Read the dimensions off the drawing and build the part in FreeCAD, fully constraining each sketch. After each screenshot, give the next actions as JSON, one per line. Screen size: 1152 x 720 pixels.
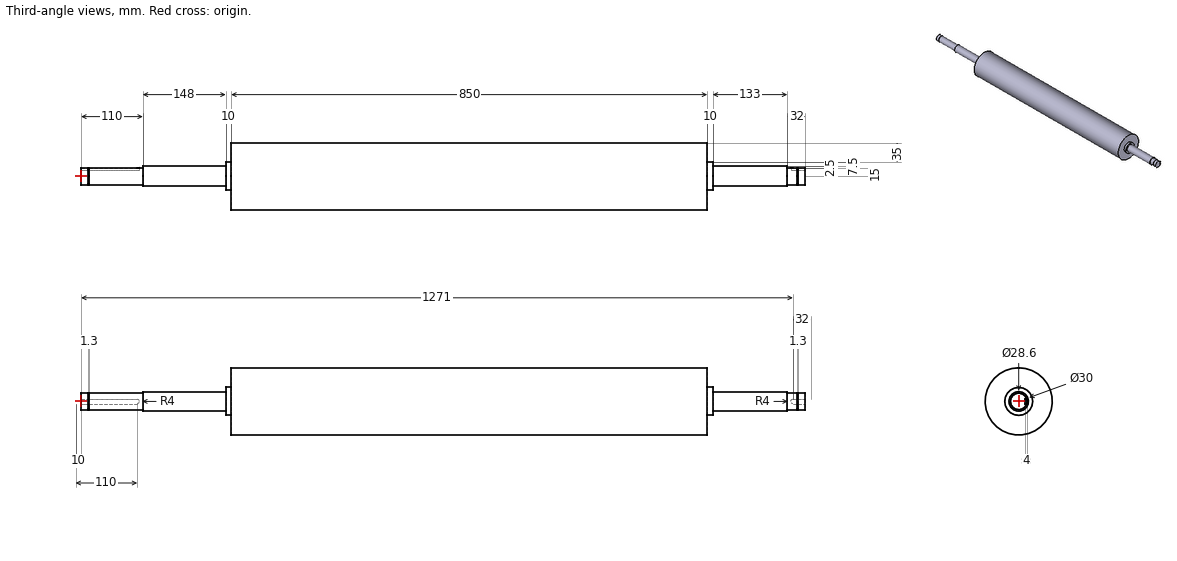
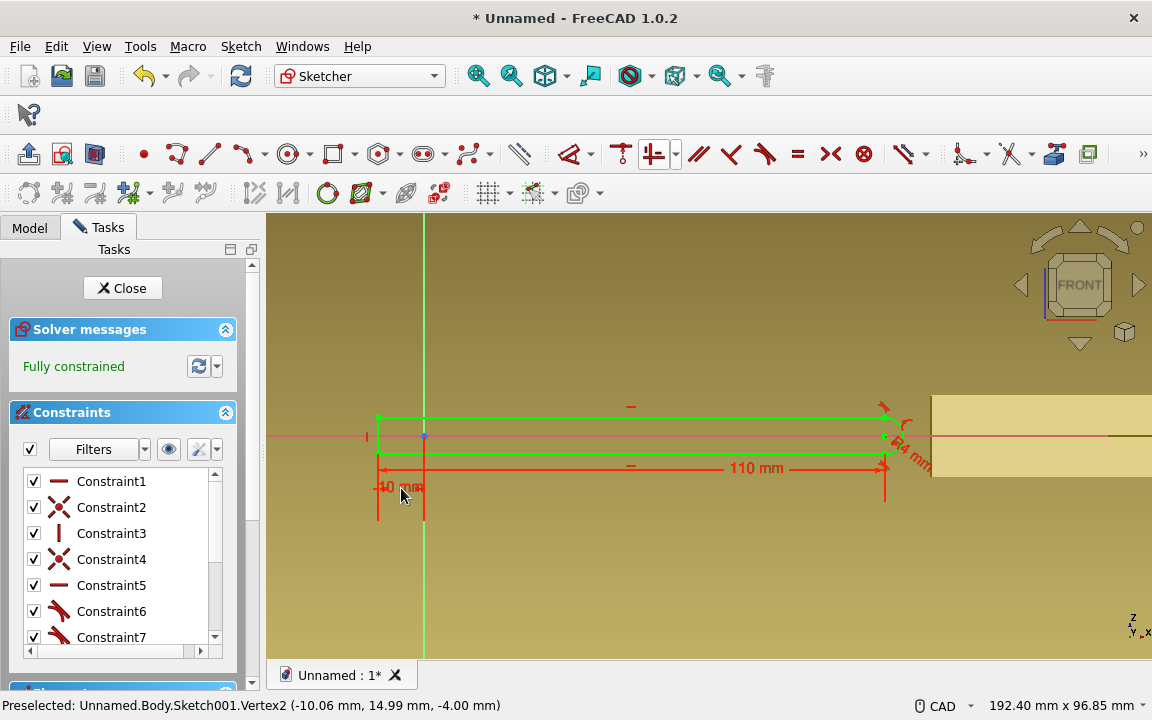
{"action": "left_click", "coordinate": [123, 288]}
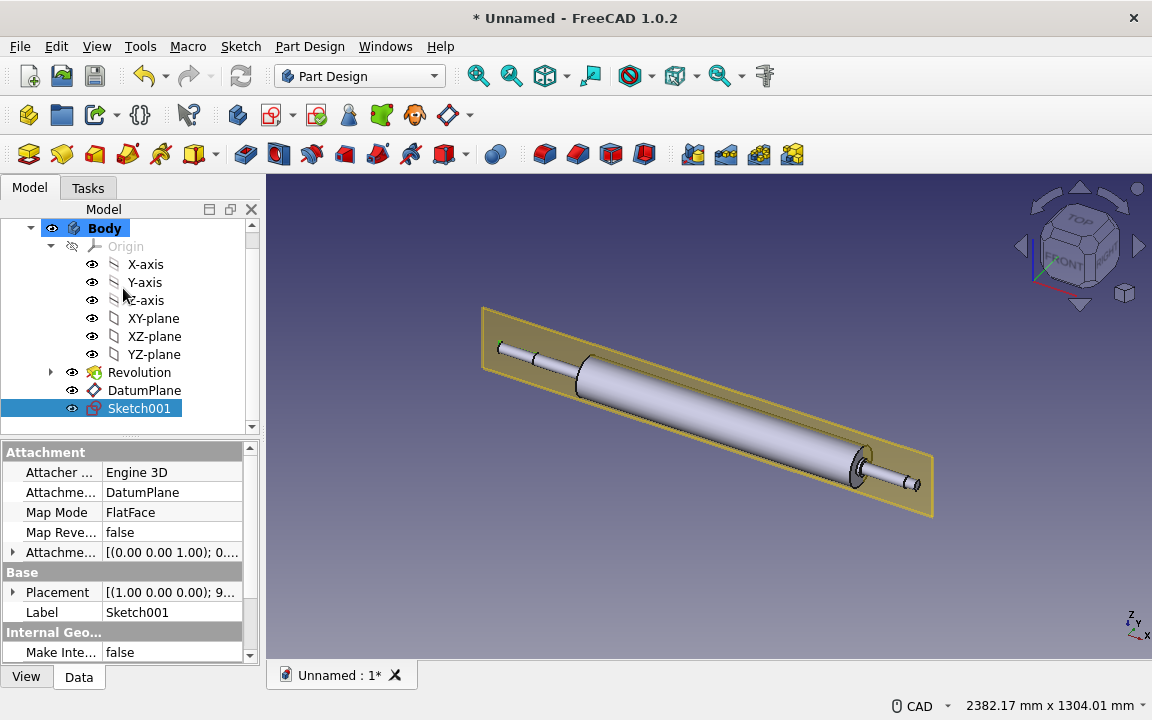
{"action": "left_click", "coordinate": [246, 154]}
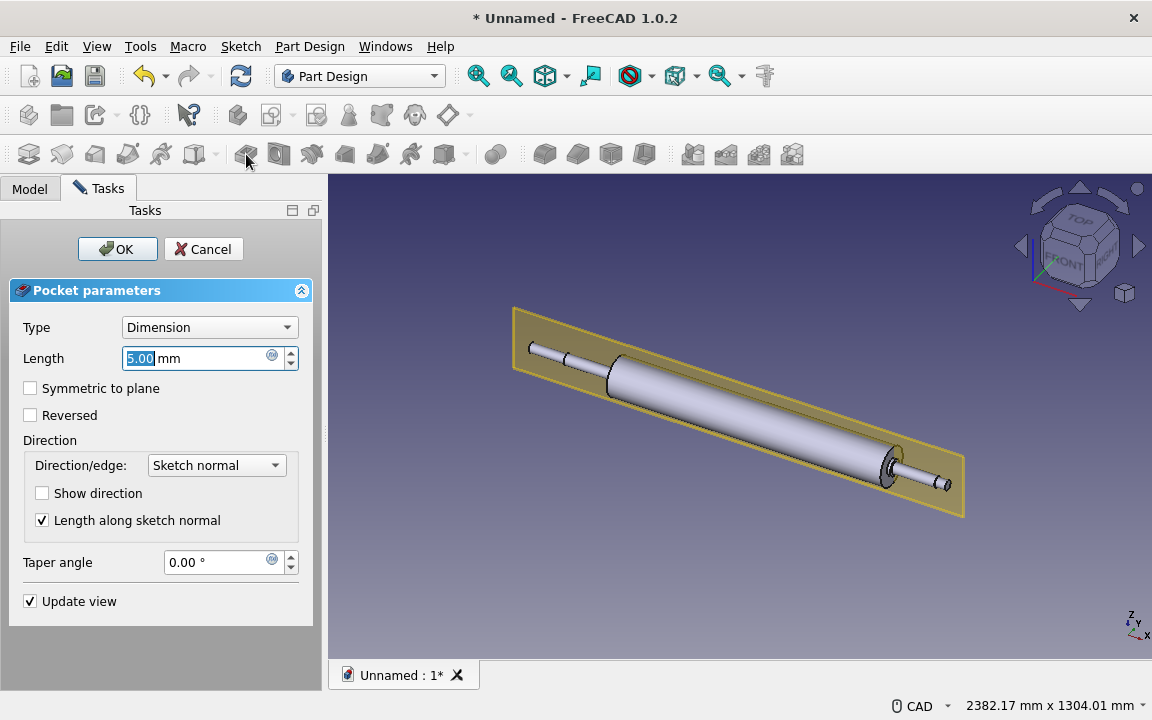
{"action": "type", "text": "4"}
{"action": "key", "text": "Tab"}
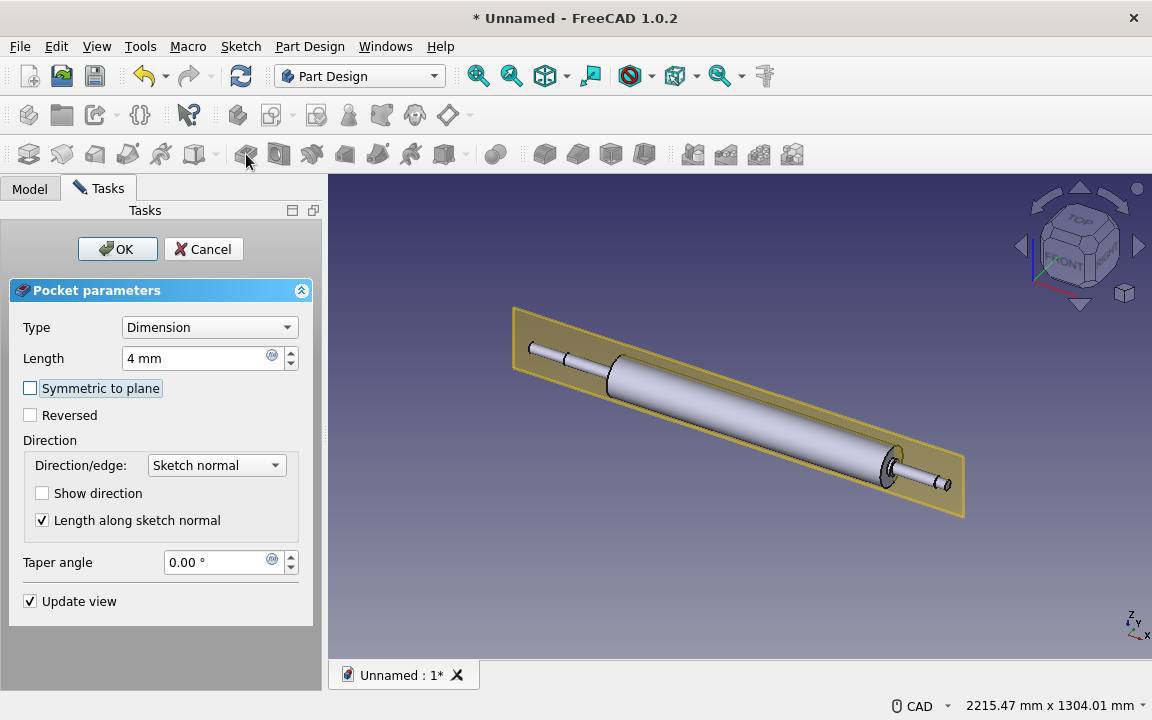
{"action": "left_click", "coordinate": [31, 415]}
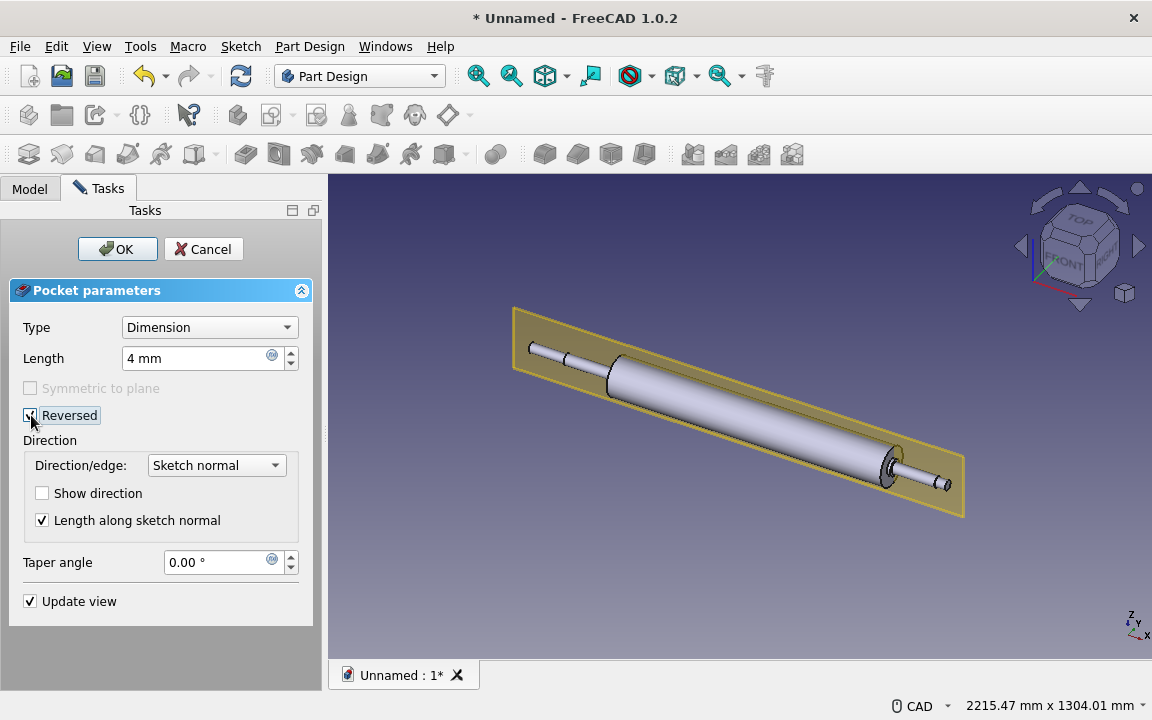
{"action": "left_click", "coordinate": [118, 249]}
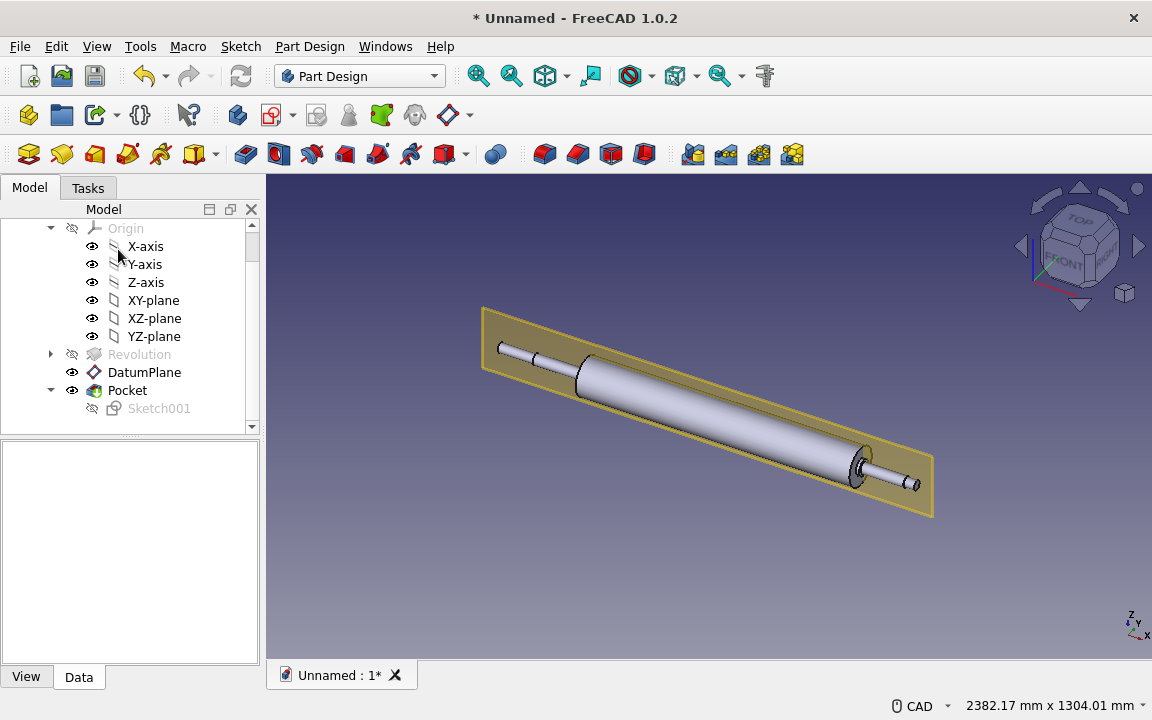
{"action": "left_click", "coordinate": [117, 372]}
{"action": "key", "text": "space"}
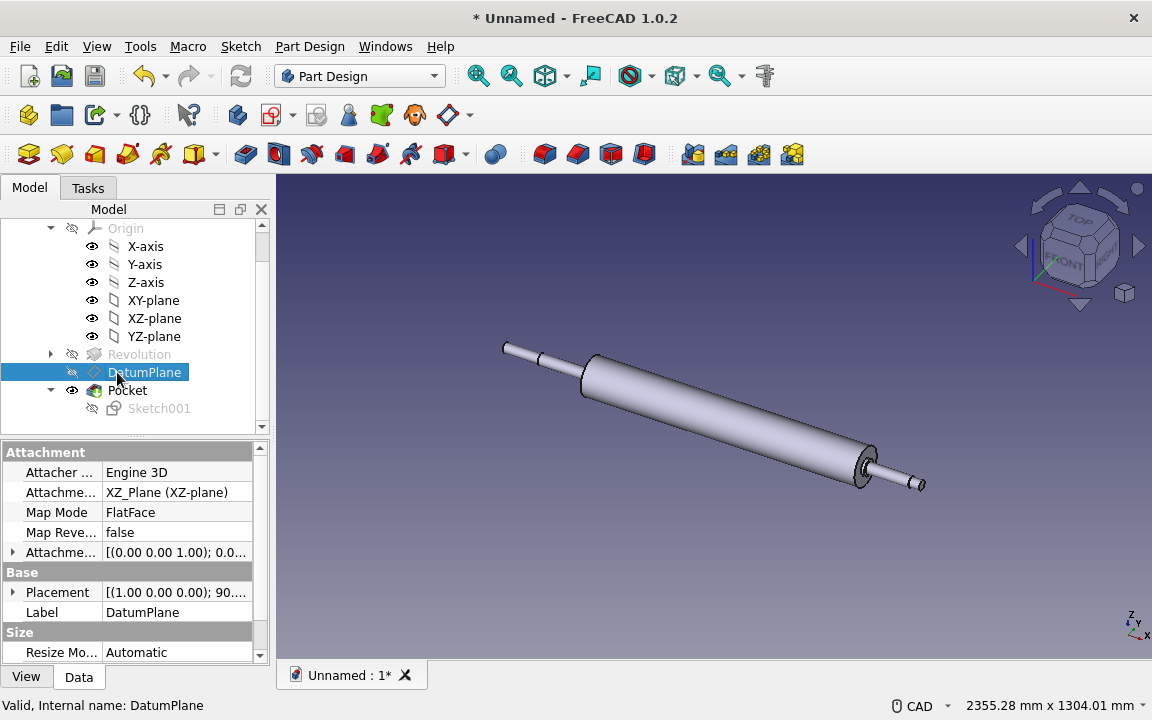
{"action": "left_click", "coordinate": [137, 336]}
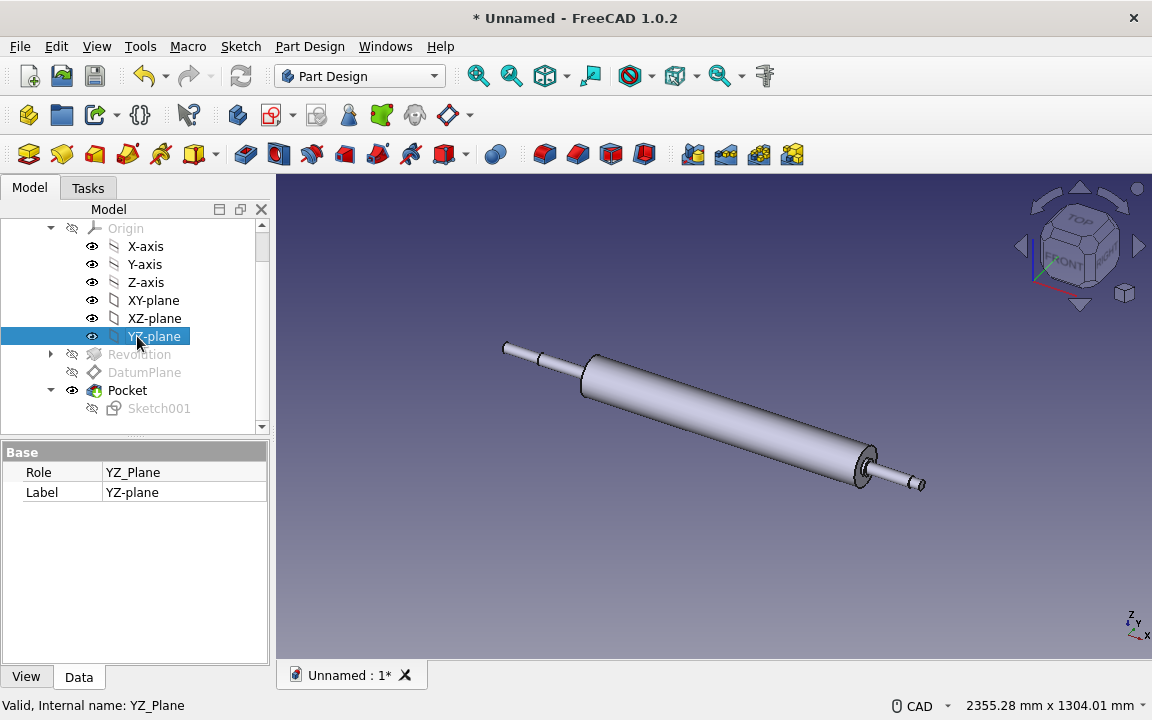
{"action": "left_click", "coordinate": [448, 116]}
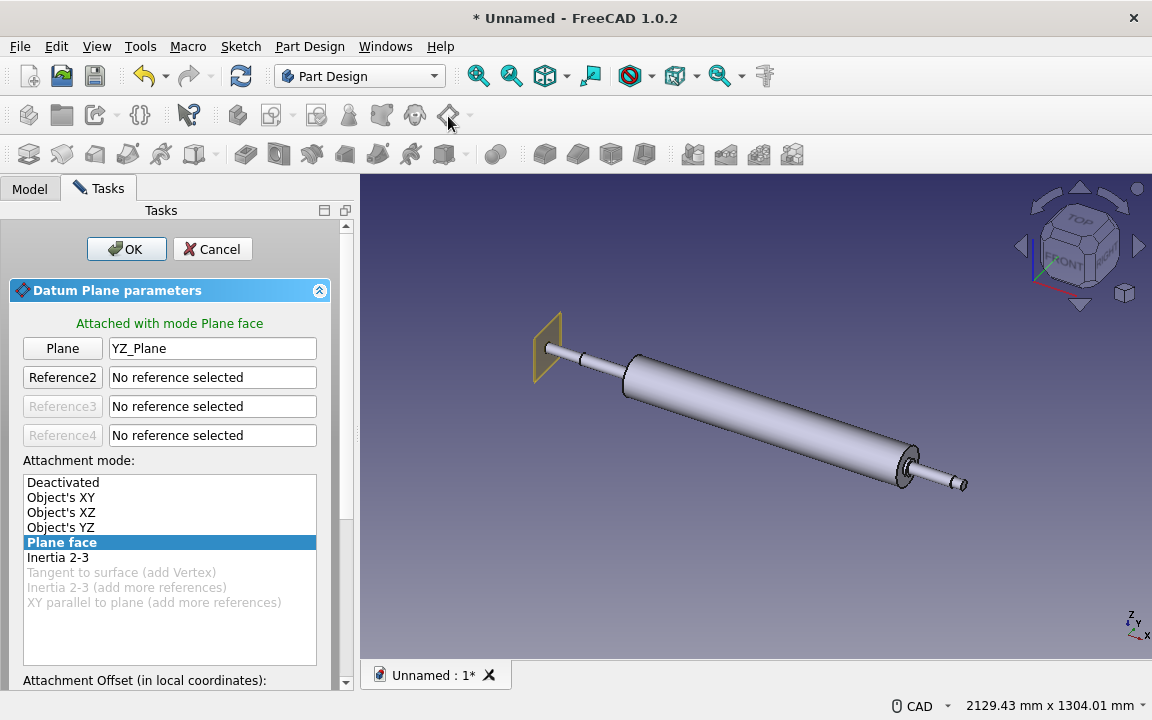
{"action": "scroll", "coordinate": [346, 455], "scroll_direction": "down", "scroll_amount": 3}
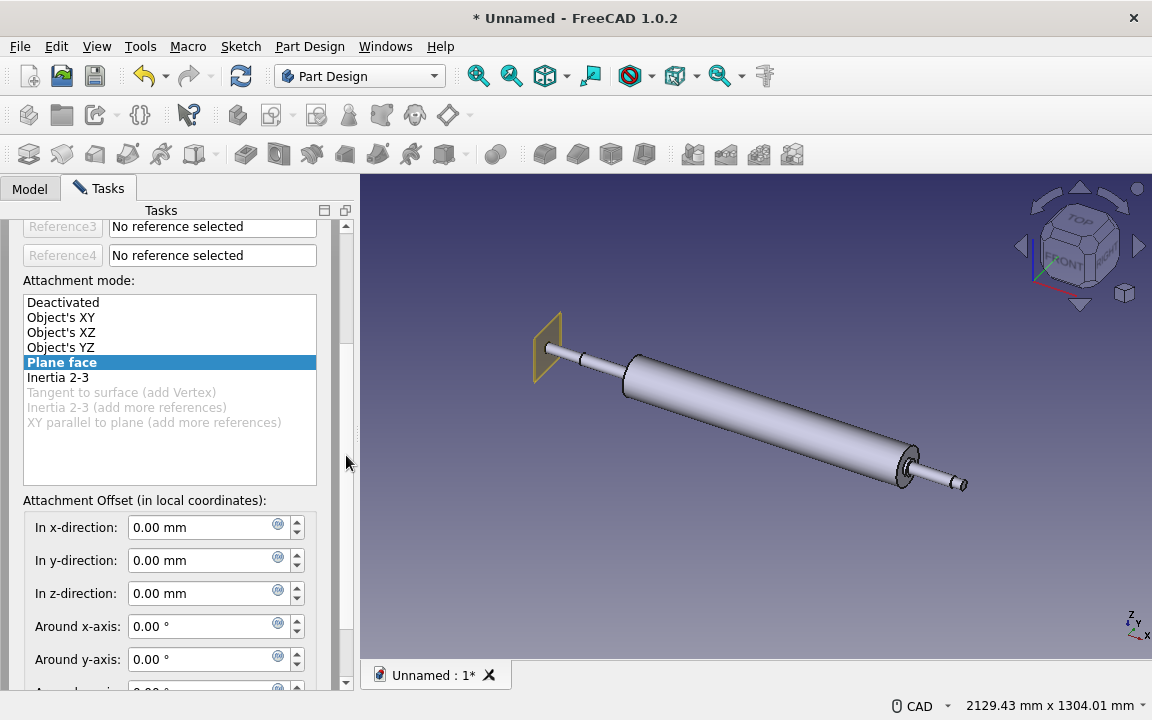
{"action": "triple_click", "coordinate": [210, 594]}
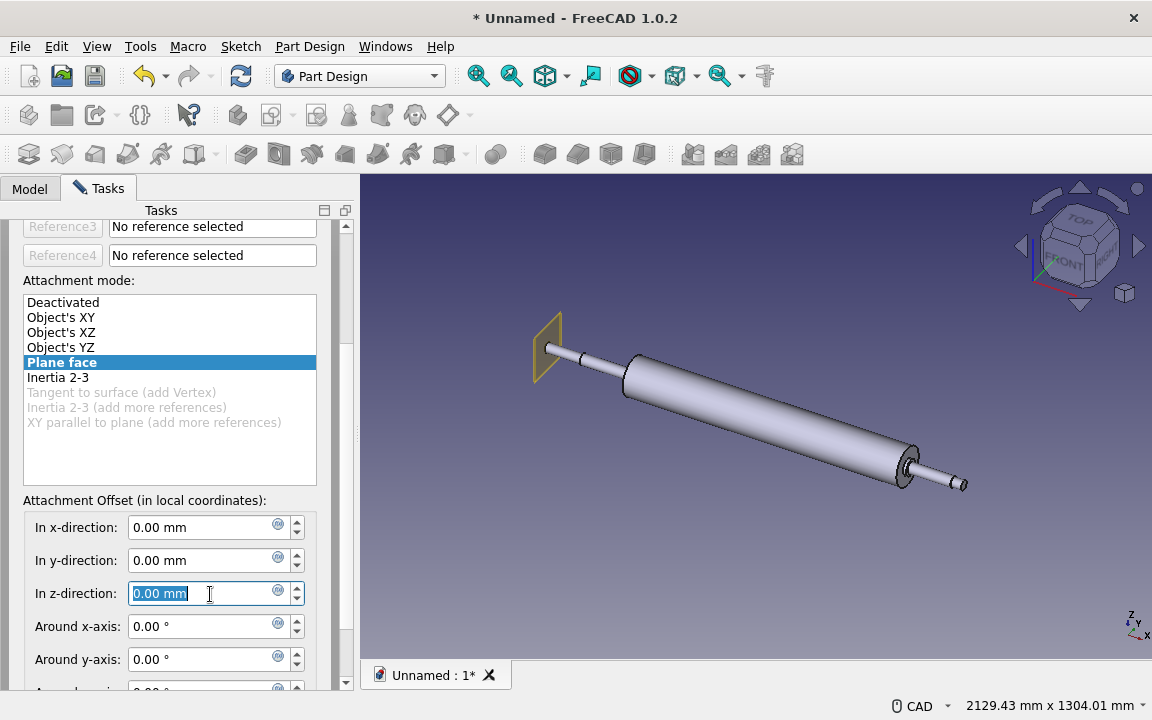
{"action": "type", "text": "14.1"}
{"action": "key", "text": "Tab"}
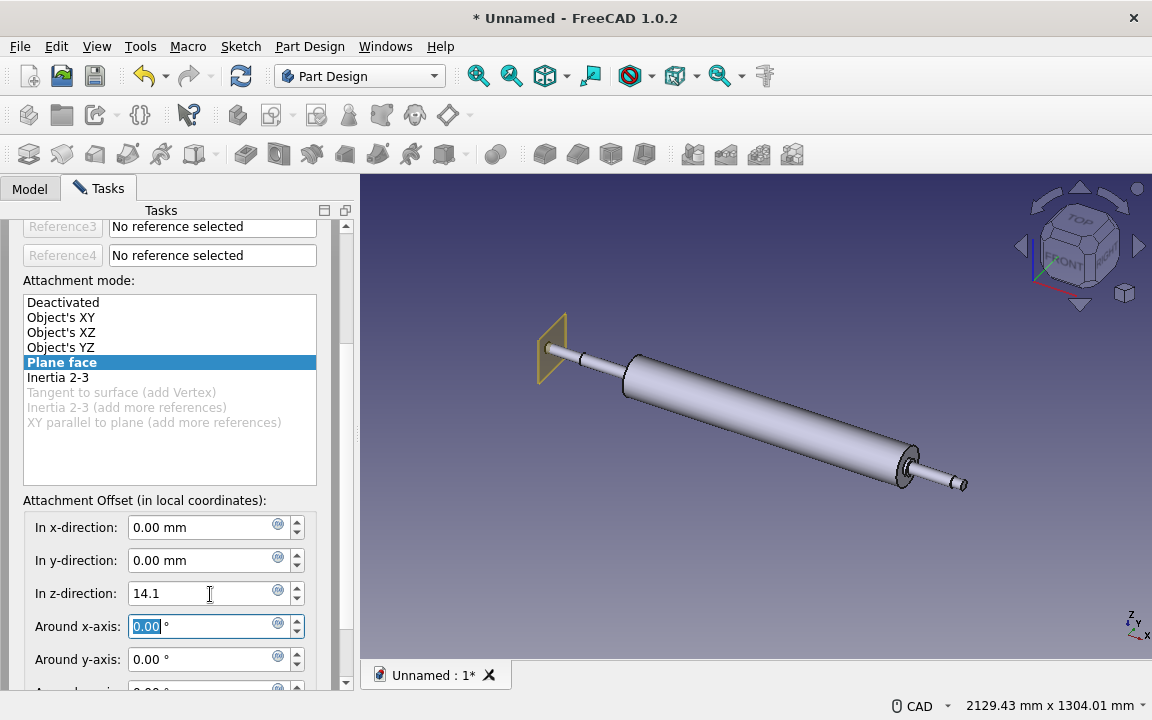
{"action": "scroll", "coordinate": [346, 455], "scroll_direction": "up", "scroll_amount": 4}